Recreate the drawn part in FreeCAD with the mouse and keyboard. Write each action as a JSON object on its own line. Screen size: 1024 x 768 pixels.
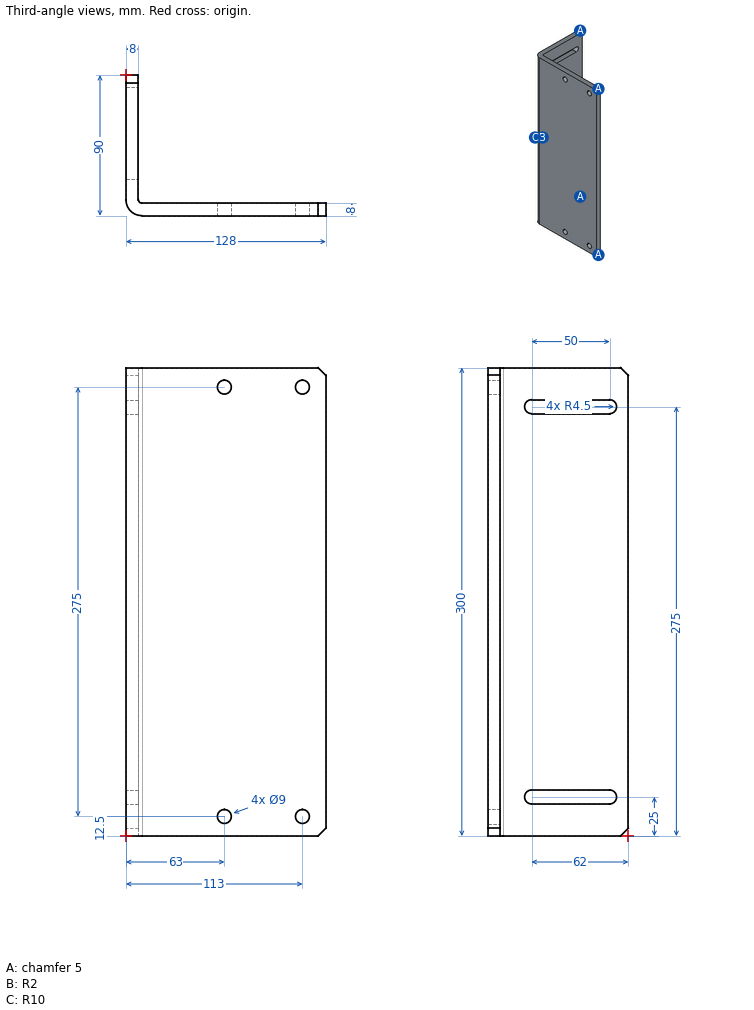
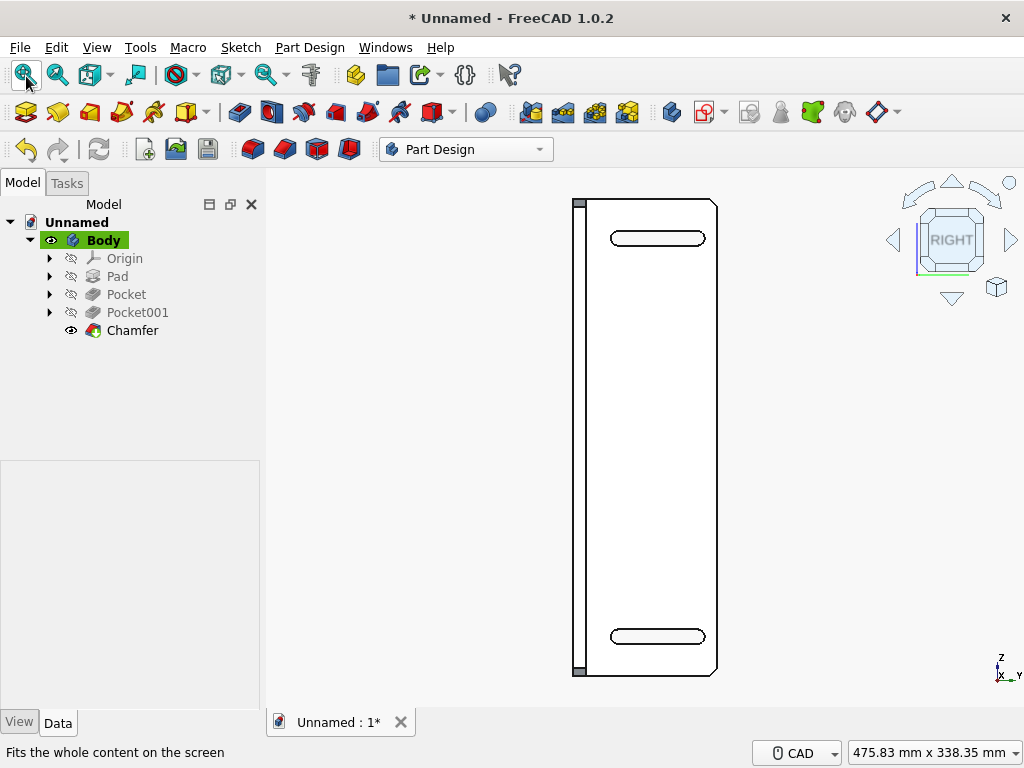
{"action": "key", "text": "5"}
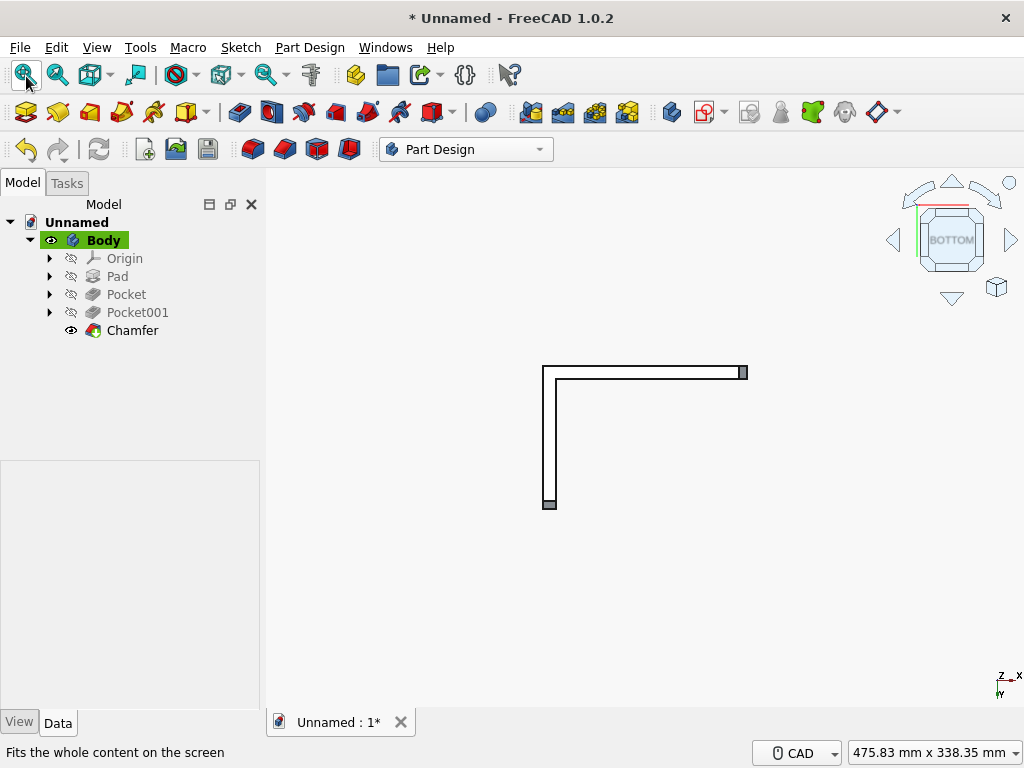
{"action": "key", "text": "v f"}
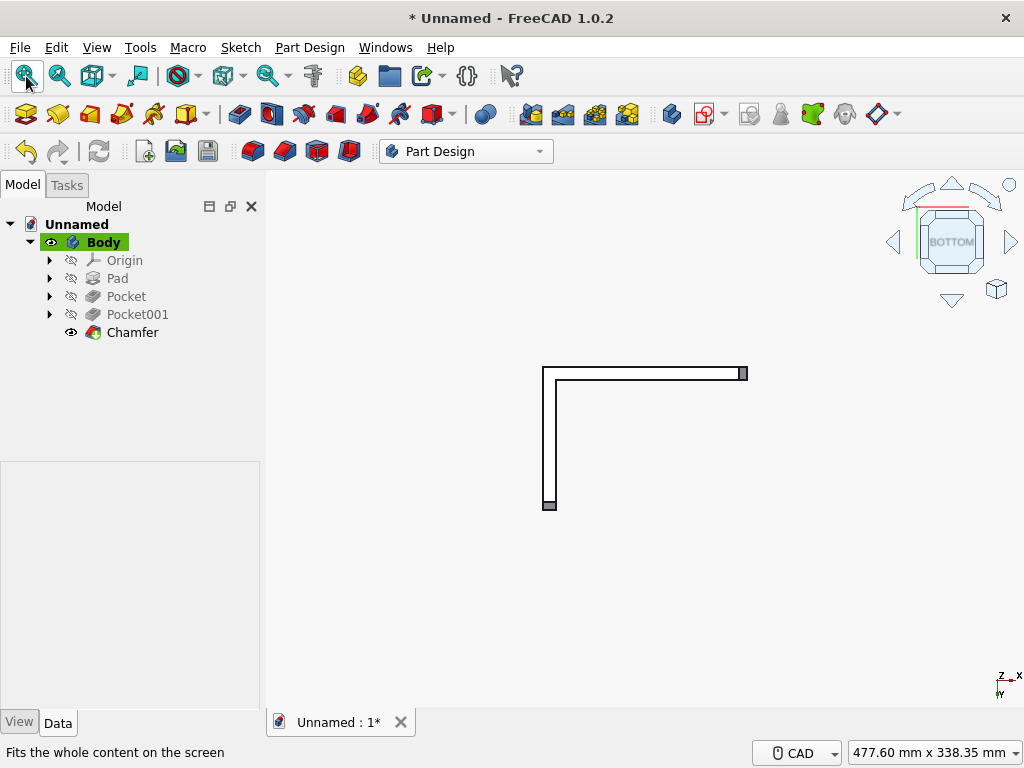
{"action": "key", "text": "4"}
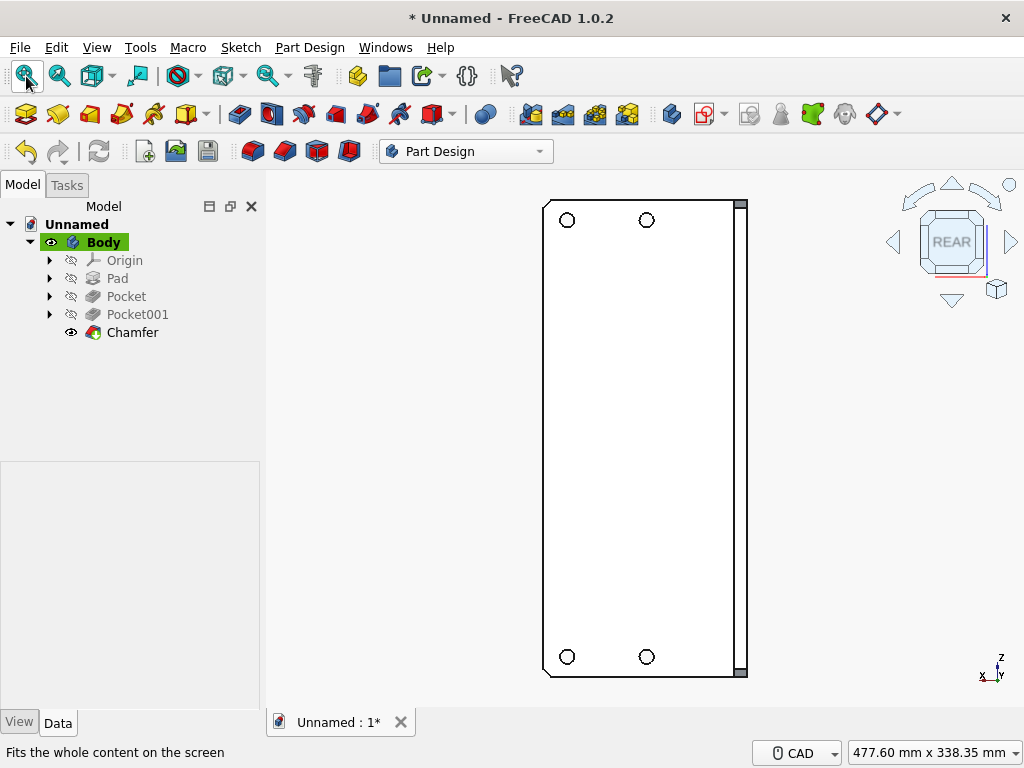
{"action": "key", "text": "6"}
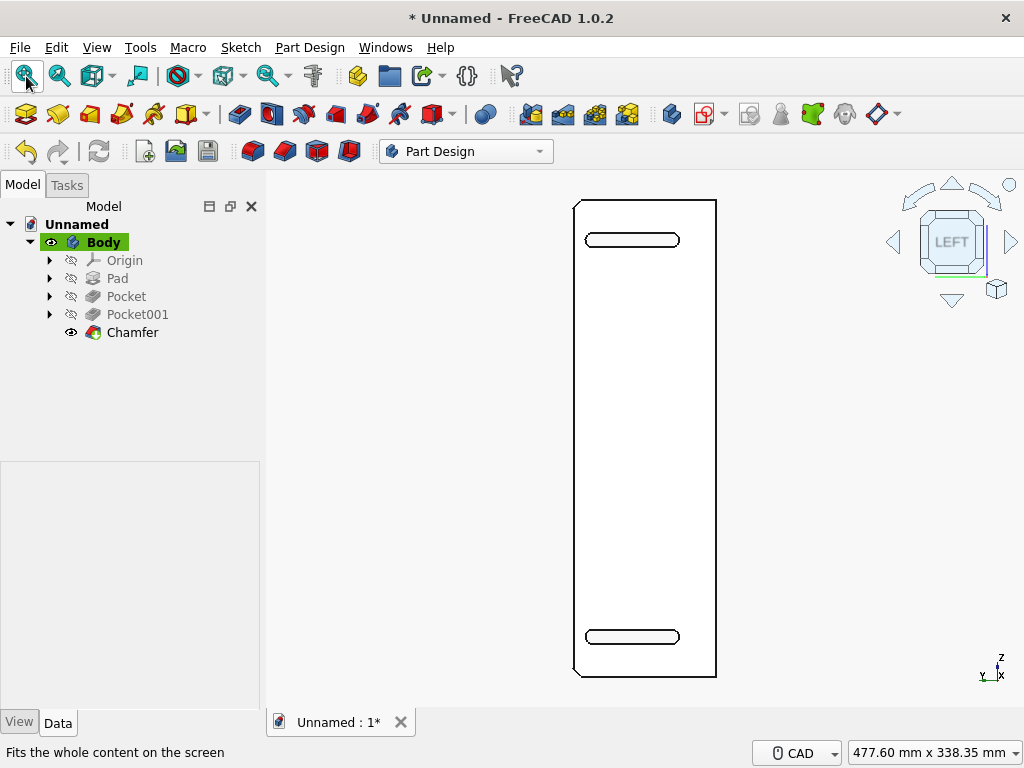
{"action": "key", "text": "v 3"}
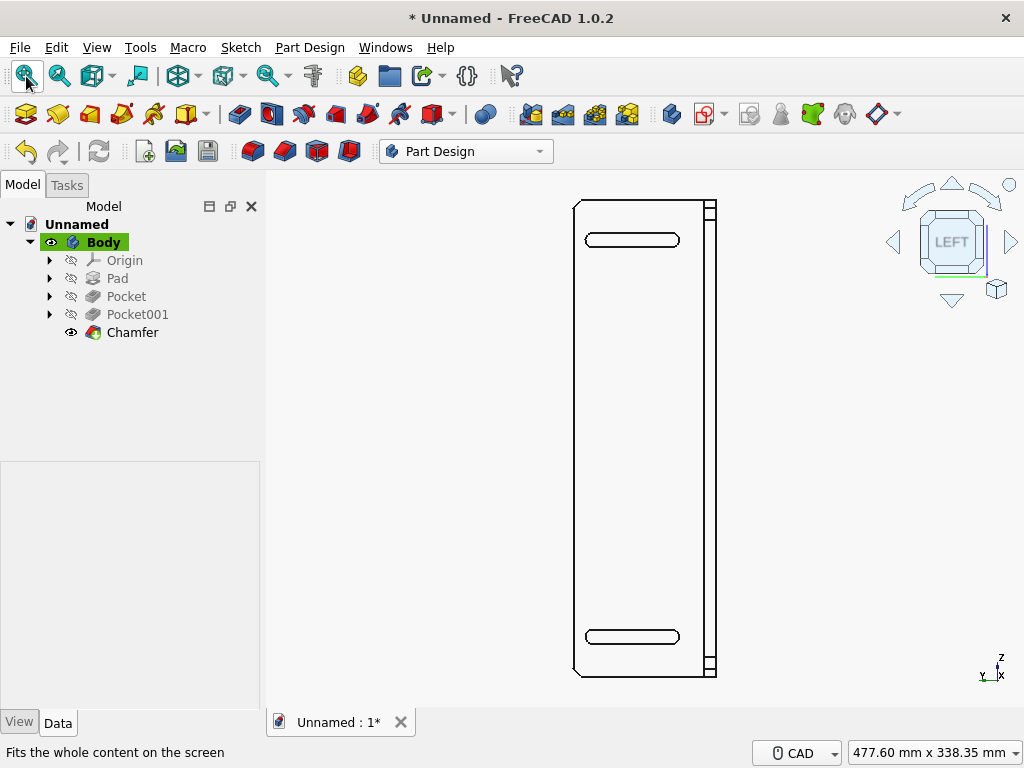
{"action": "key", "text": "0"}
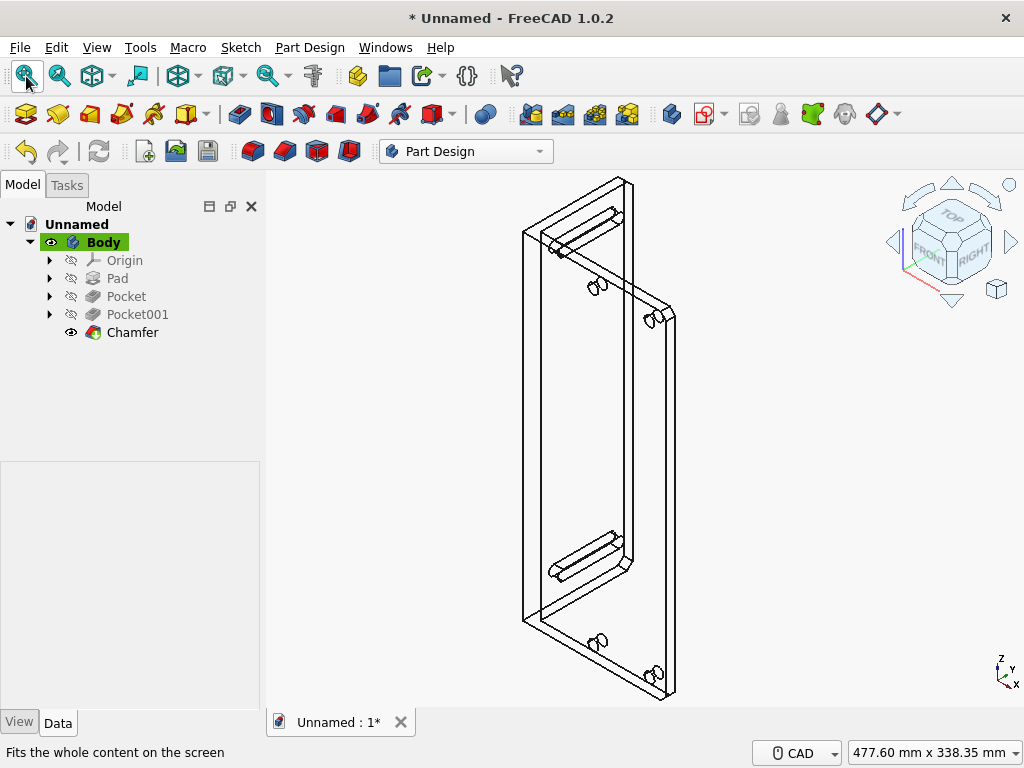
{"action": "left_click", "coordinate": [541, 425]}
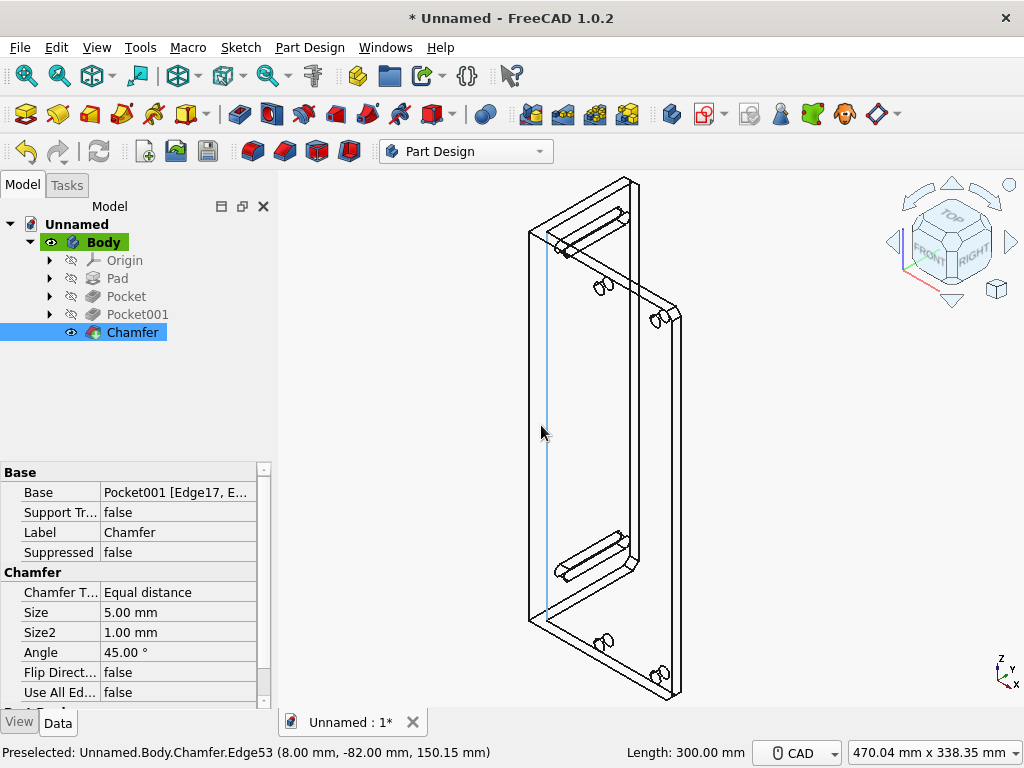
{"action": "key", "text": "v 1"}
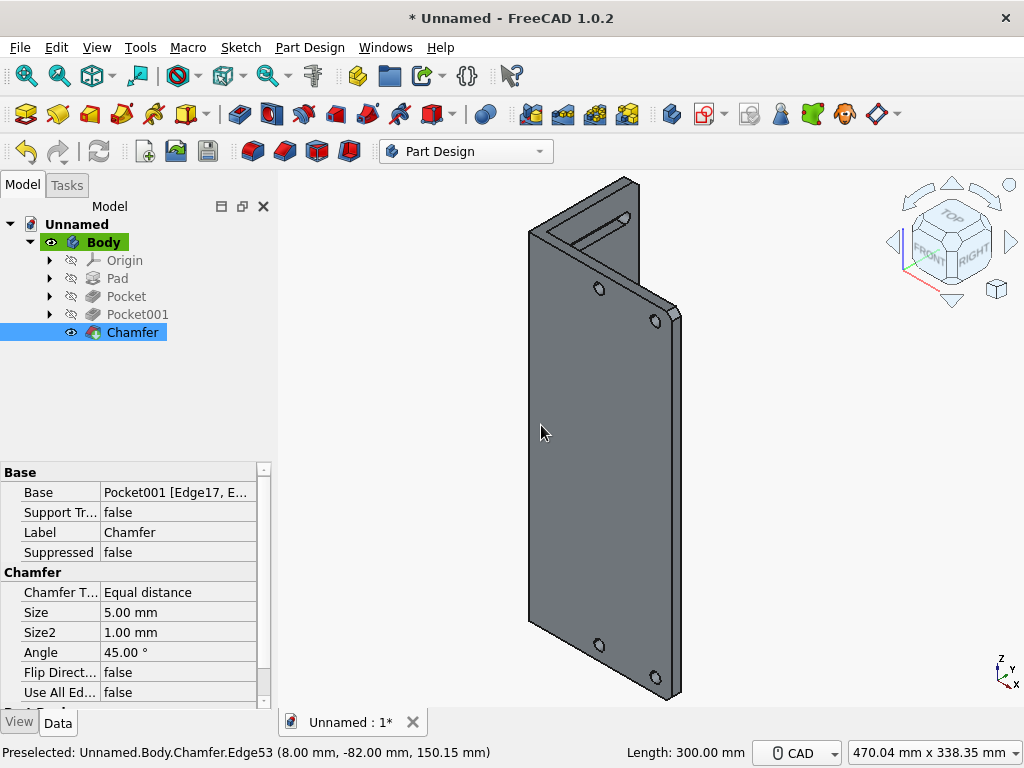
{"action": "left_click", "coordinate": [254, 152]}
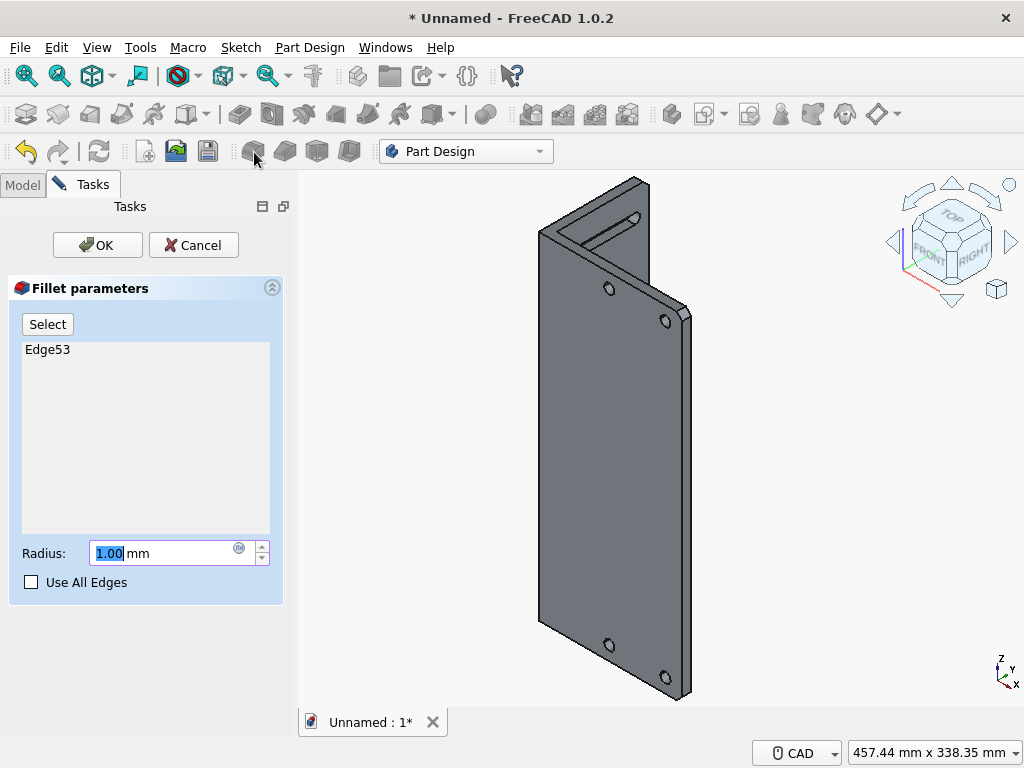
{"action": "type", "text": "2"}
{"action": "key", "text": "Tab"}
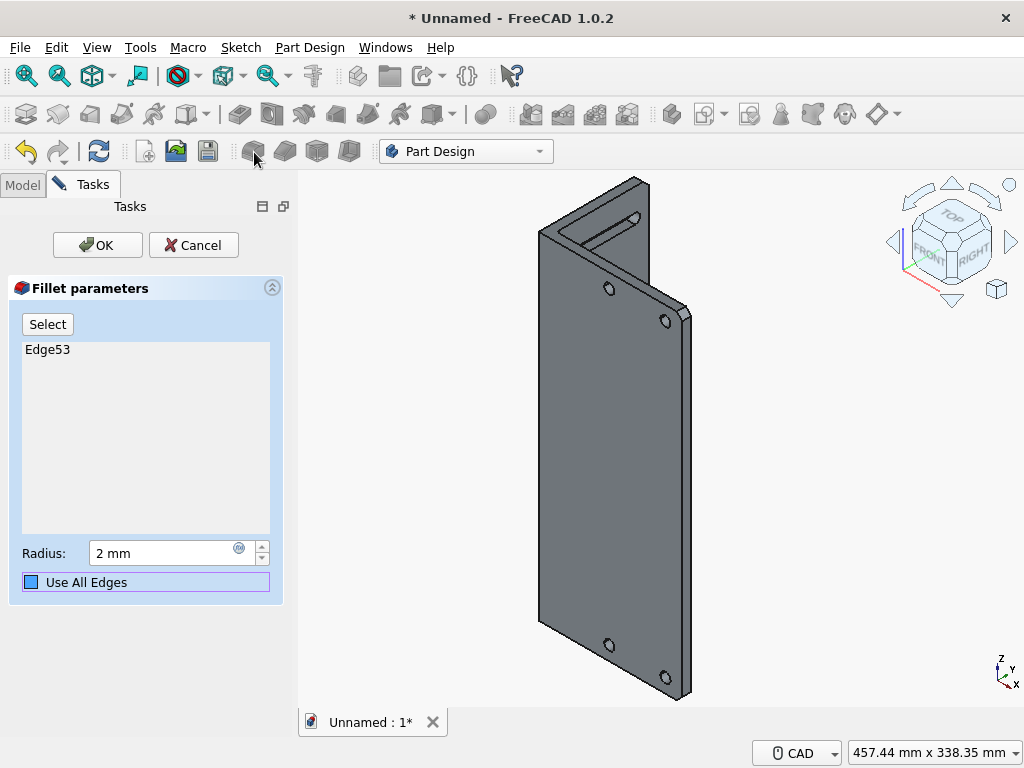
{"action": "left_click", "coordinate": [98, 245]}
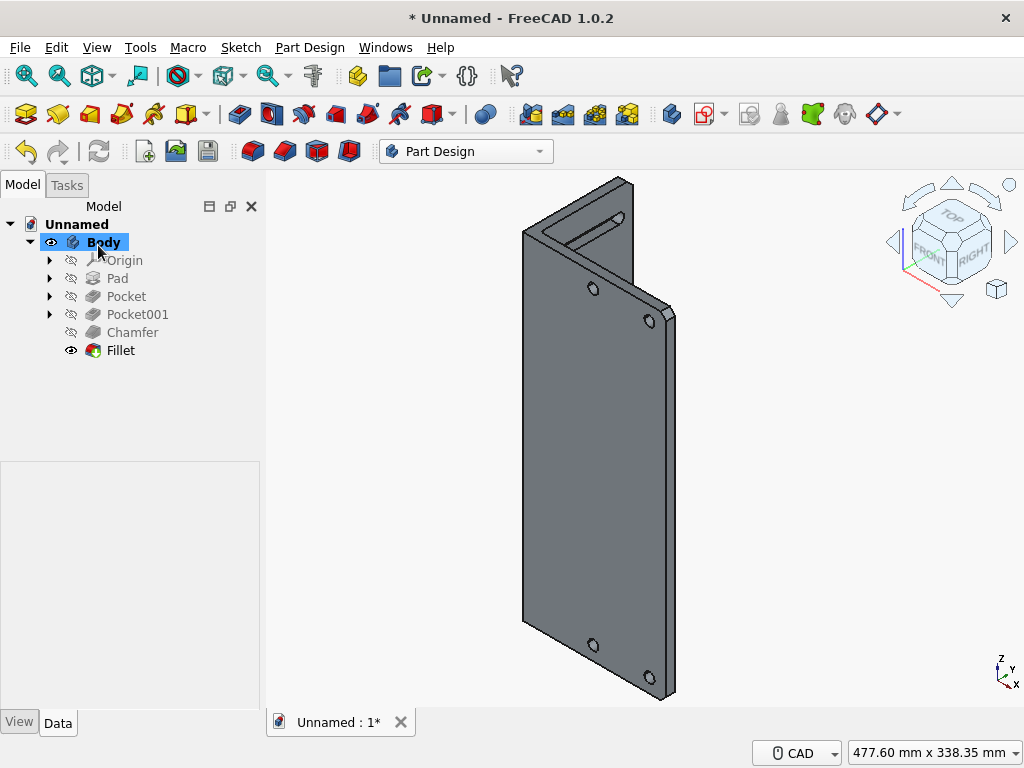
{"action": "key", "text": "2"}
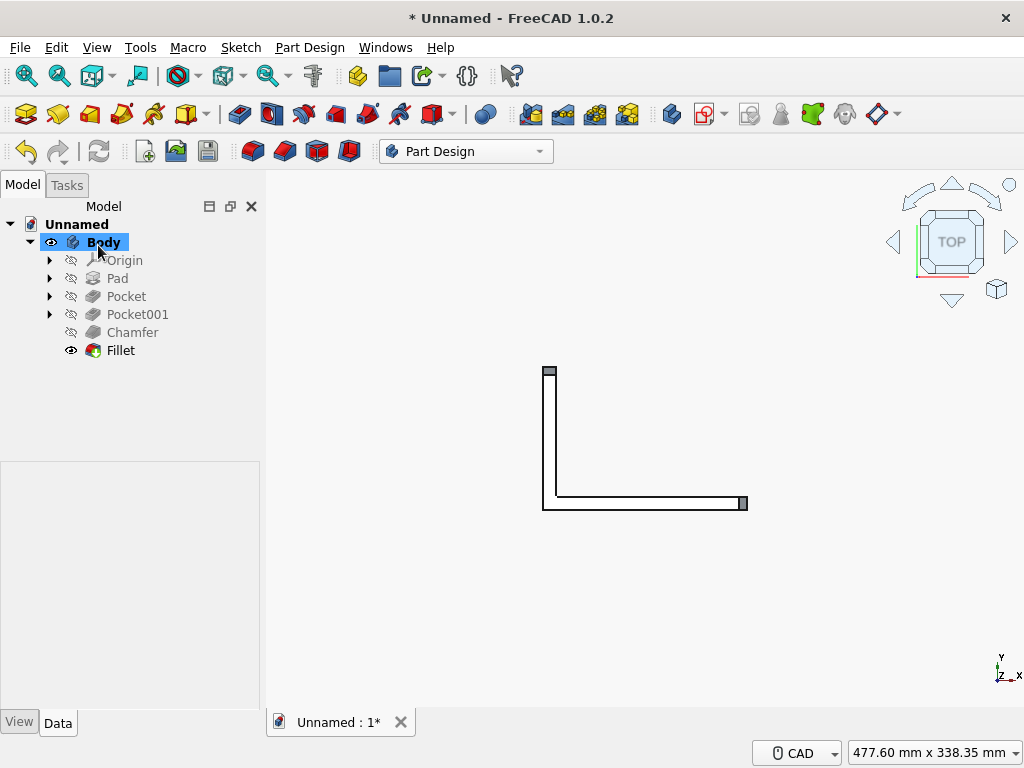
{"action": "key", "text": "v f"}